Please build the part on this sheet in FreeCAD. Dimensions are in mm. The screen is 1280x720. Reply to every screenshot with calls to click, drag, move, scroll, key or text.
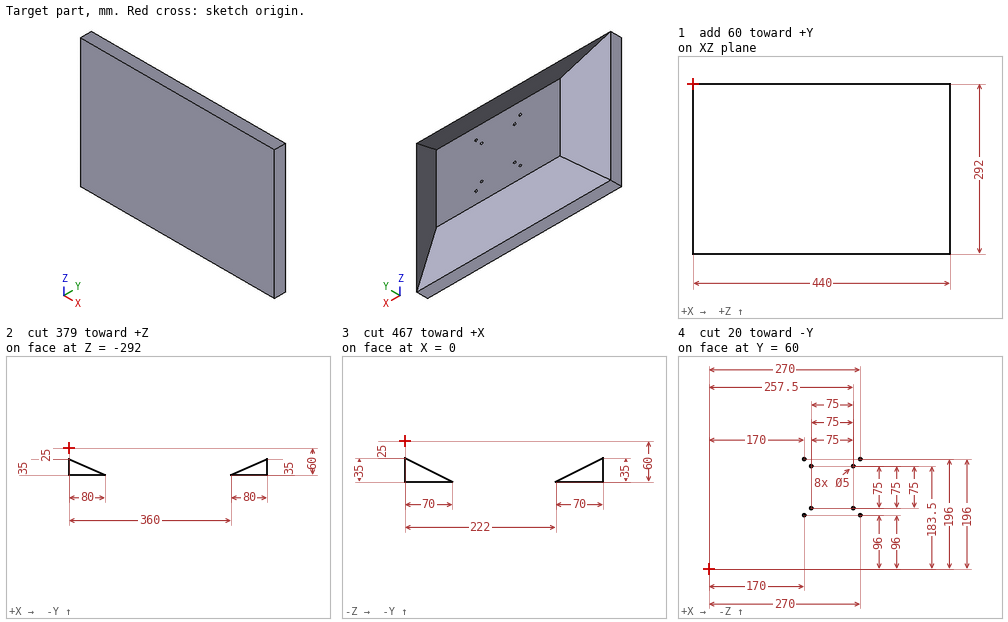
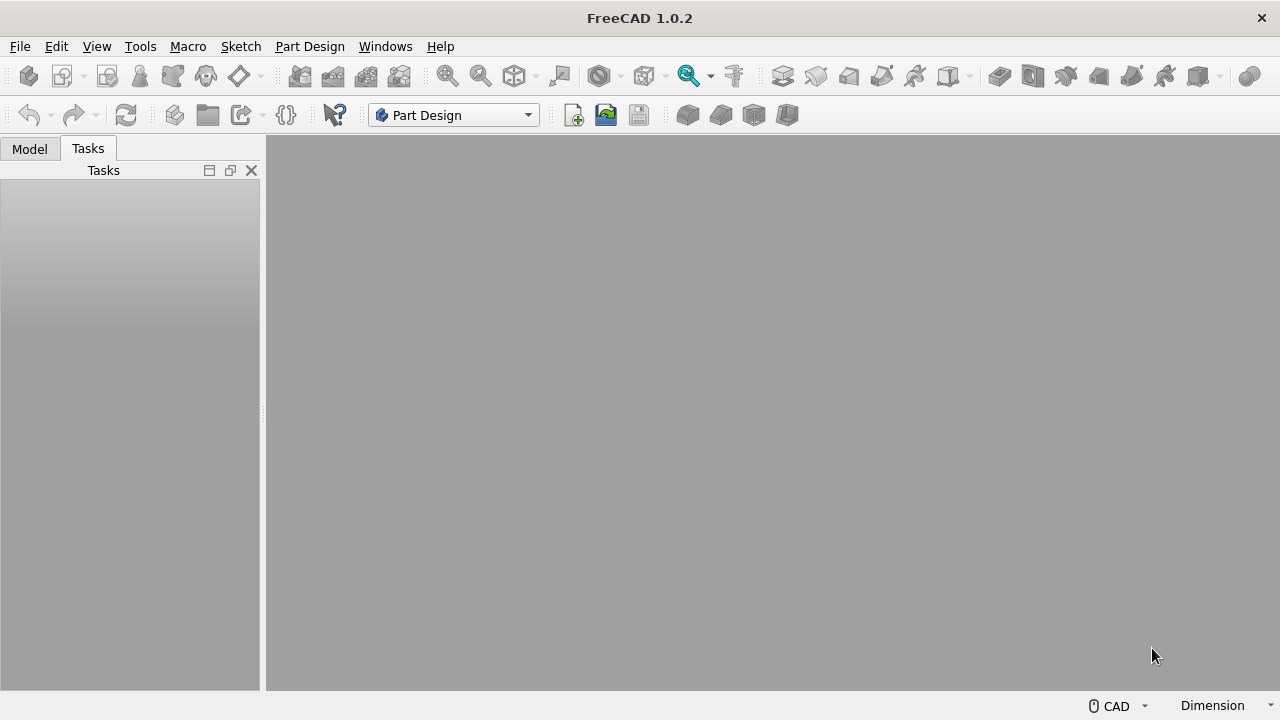
key(ctrl+n)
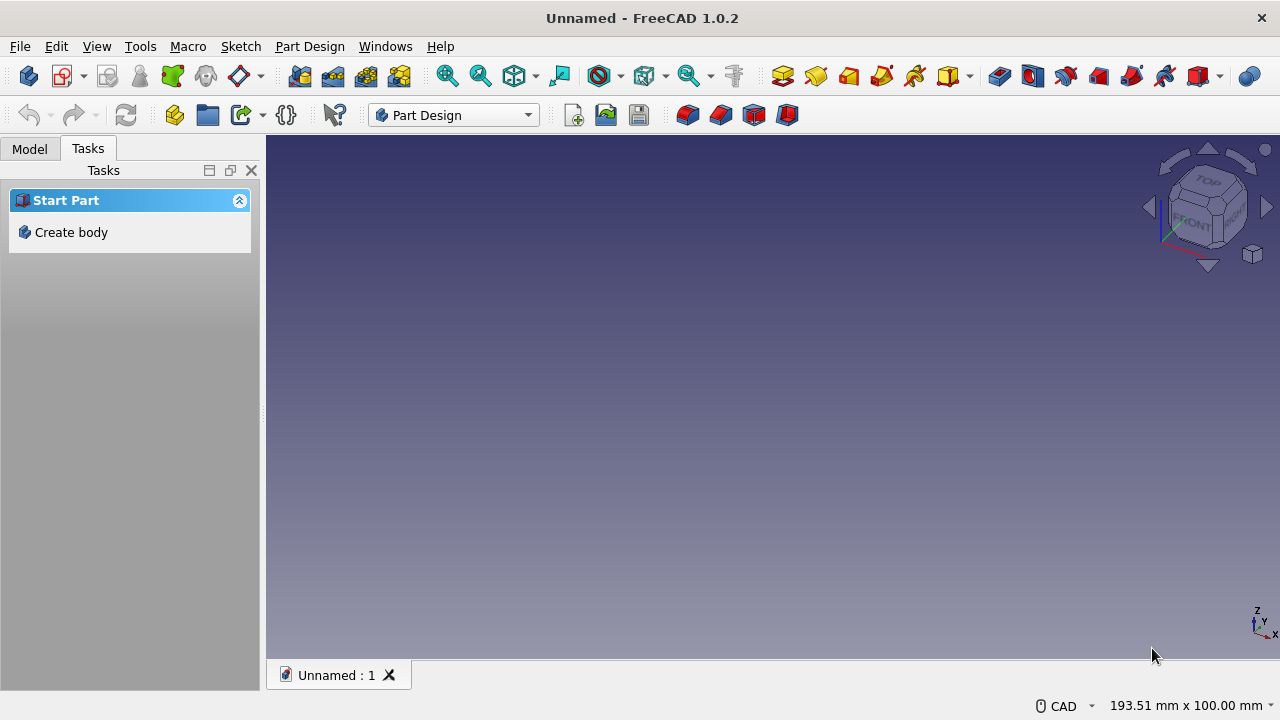
click(62, 76)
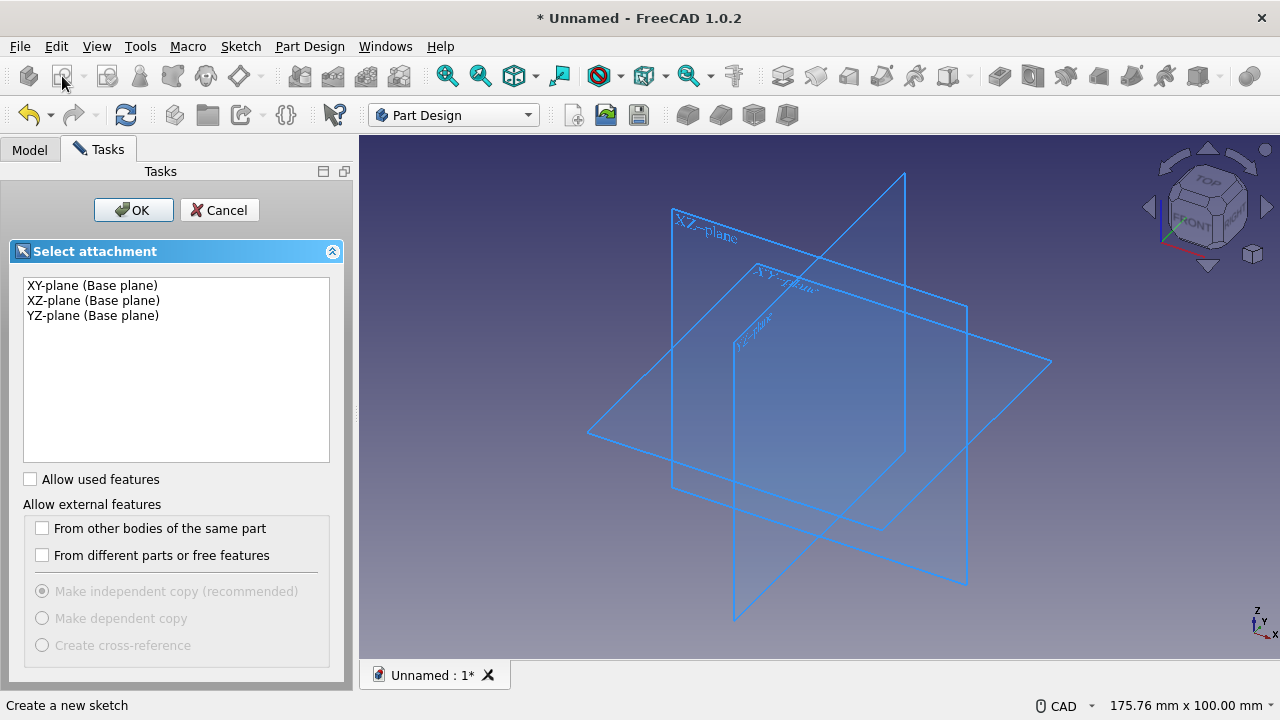
click(84, 300)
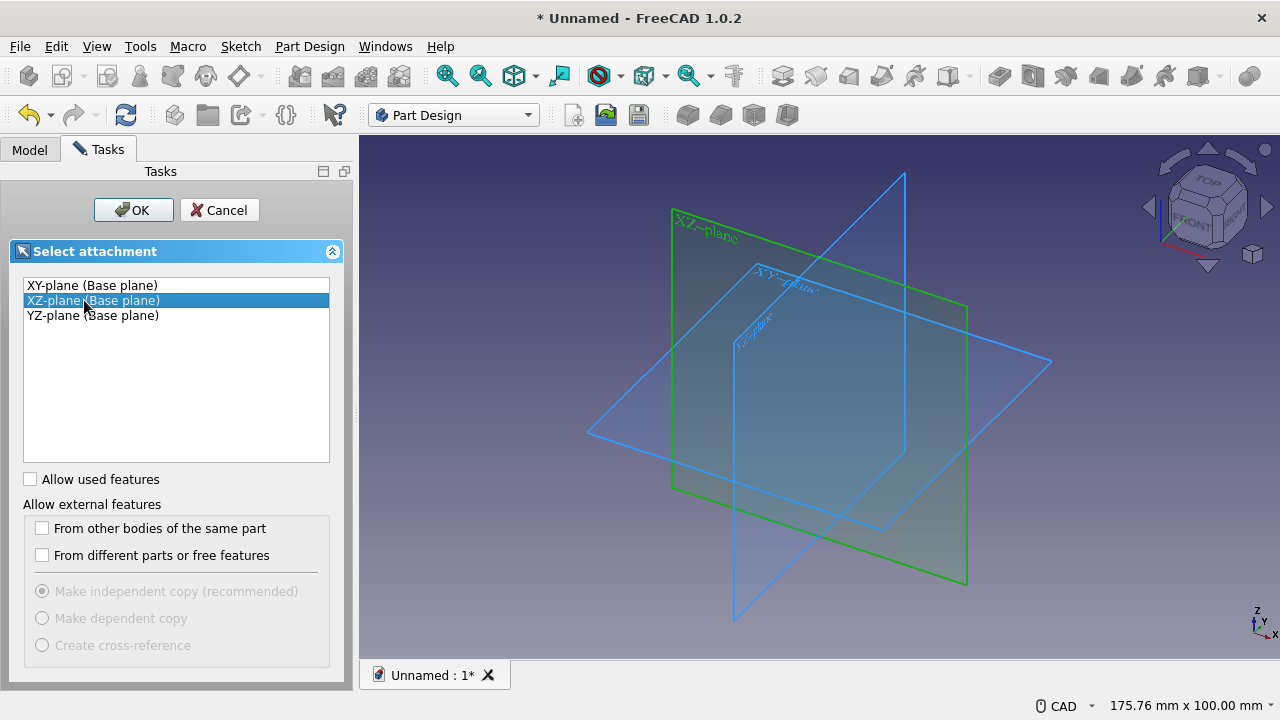
click(134, 210)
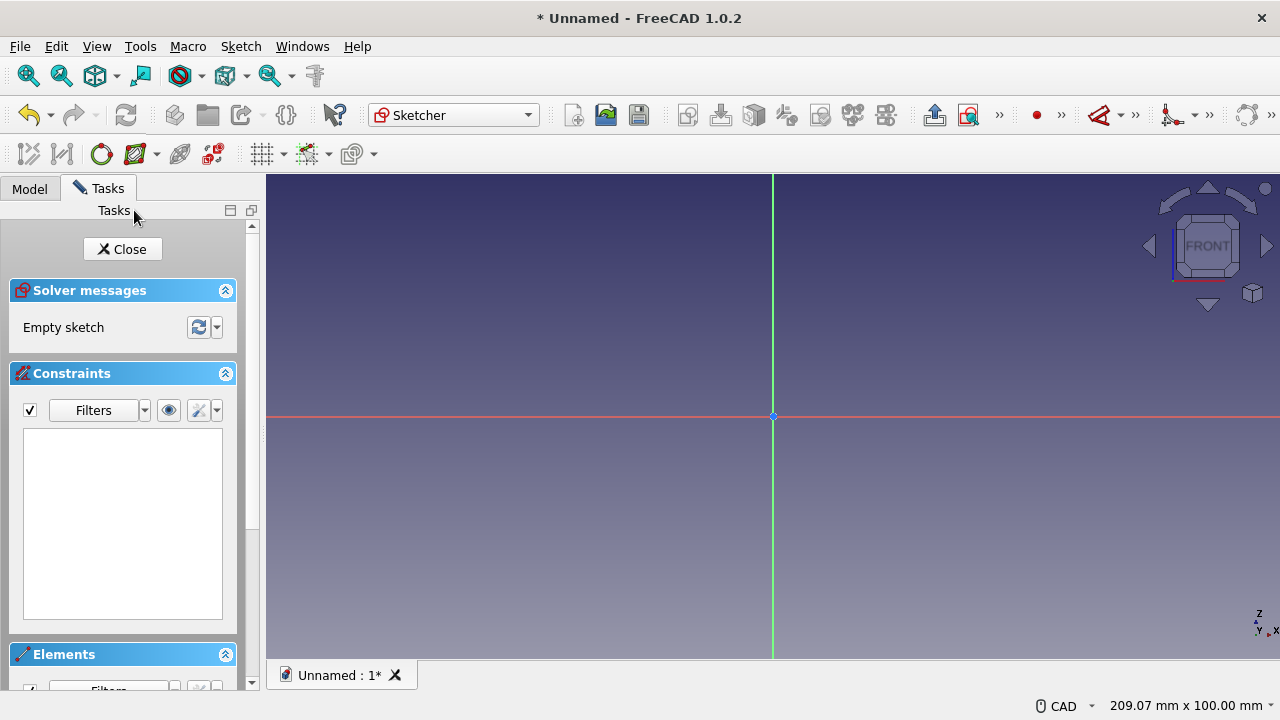
scroll(417, 237, down, 8)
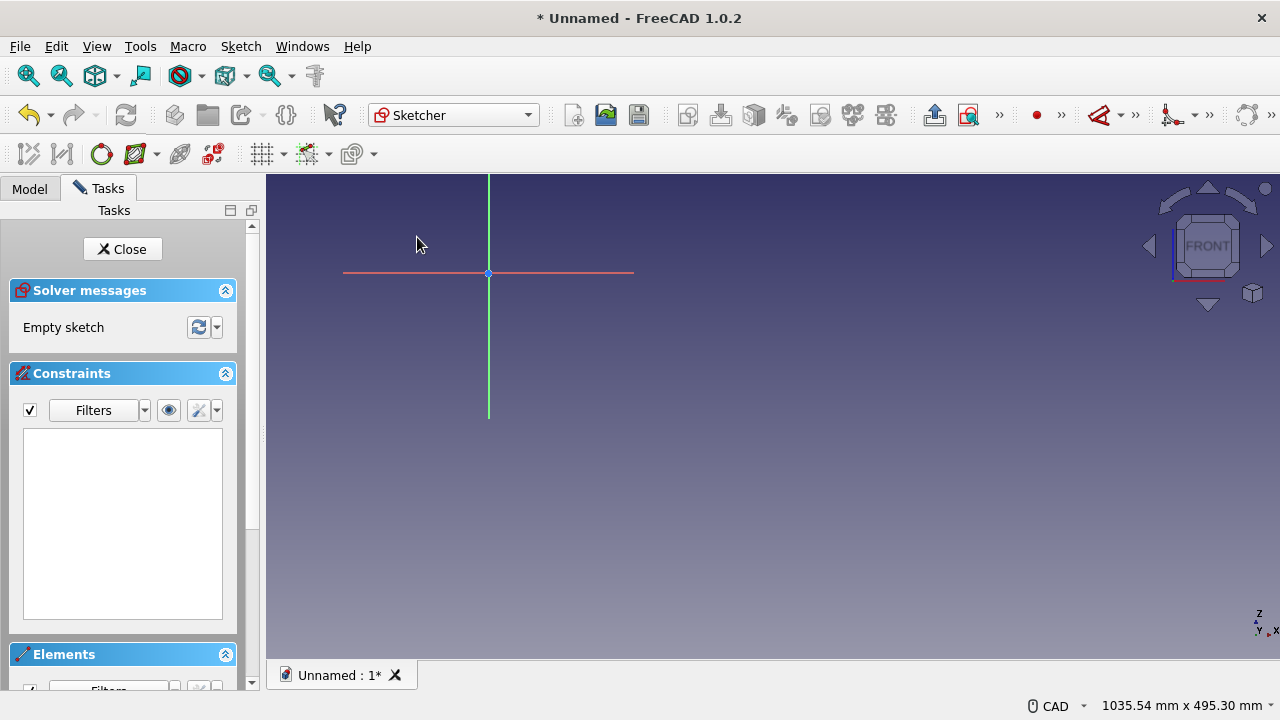
key(g)
key(r)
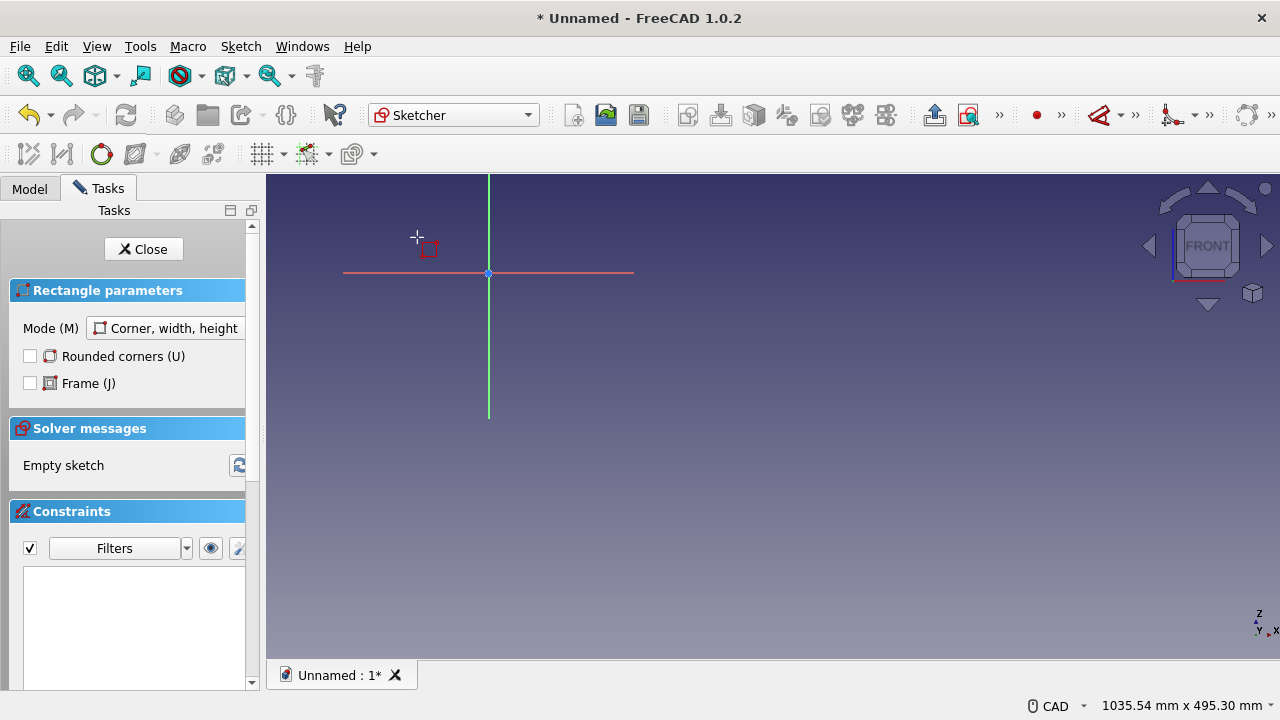
click(489, 273)
move(920, 559)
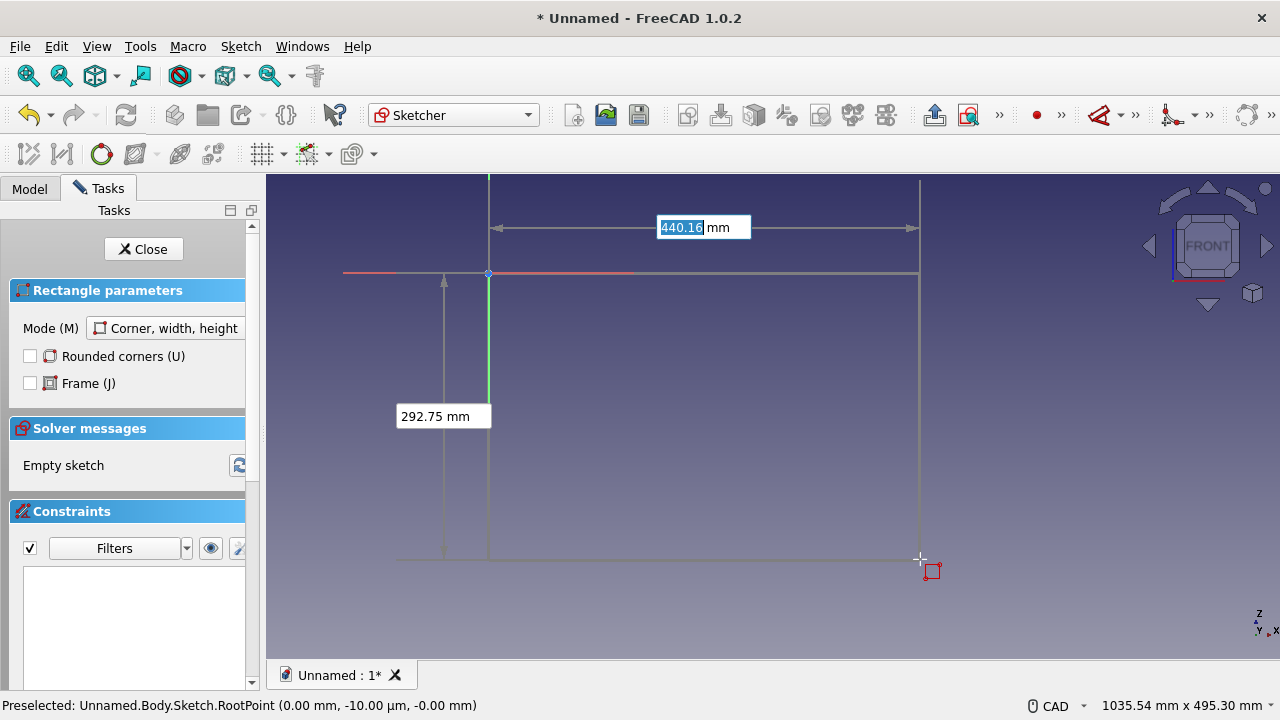
text(440)
key(Tab)
text(292)
key(Return)
key(Escape)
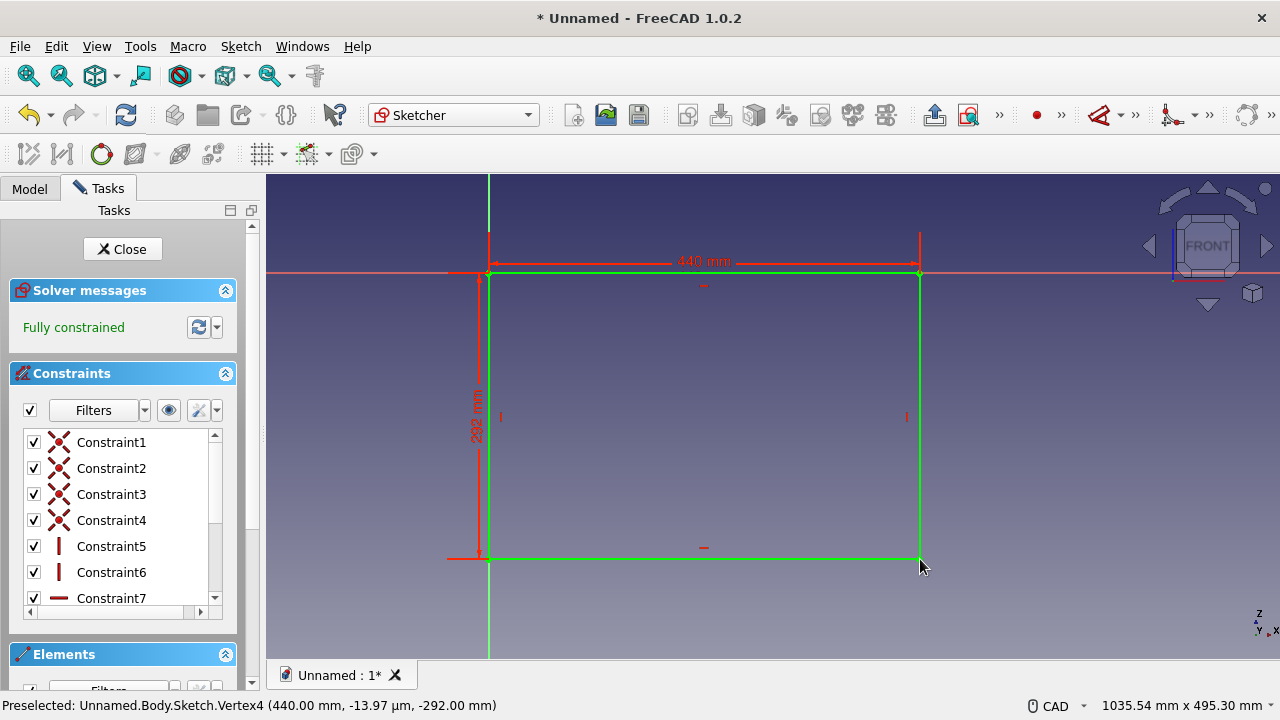
click(123, 249)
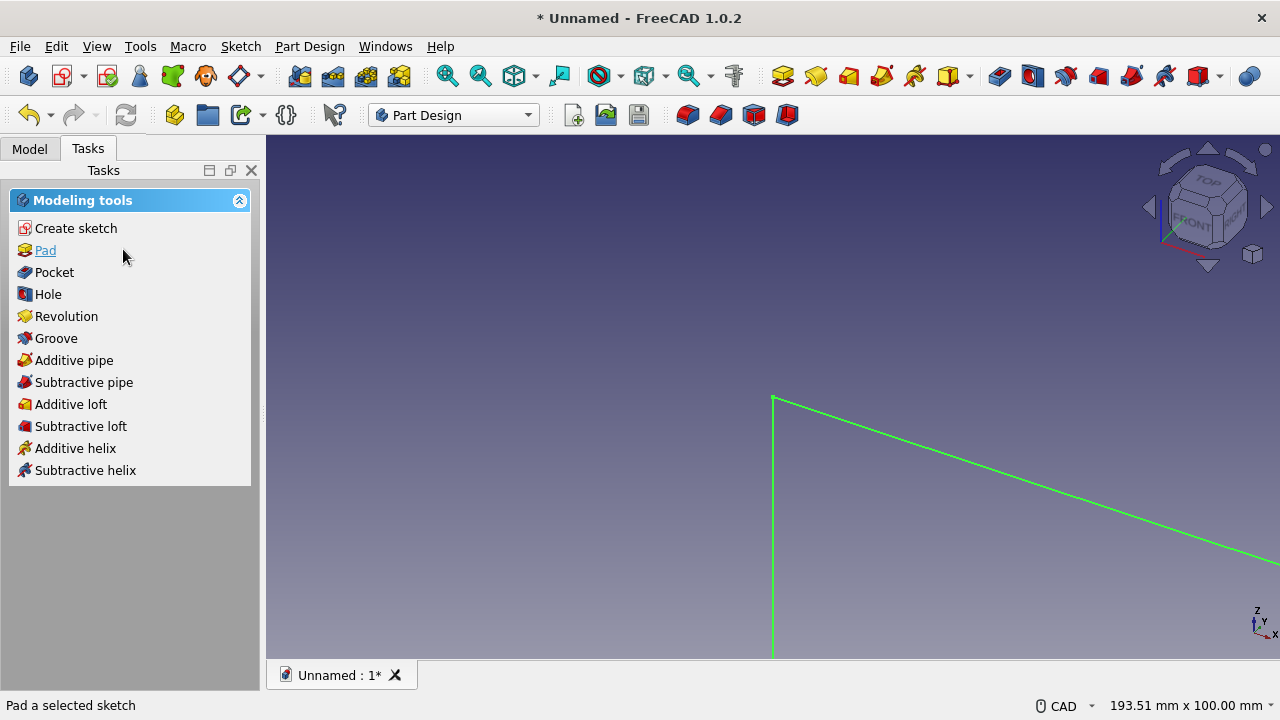
click(783, 76)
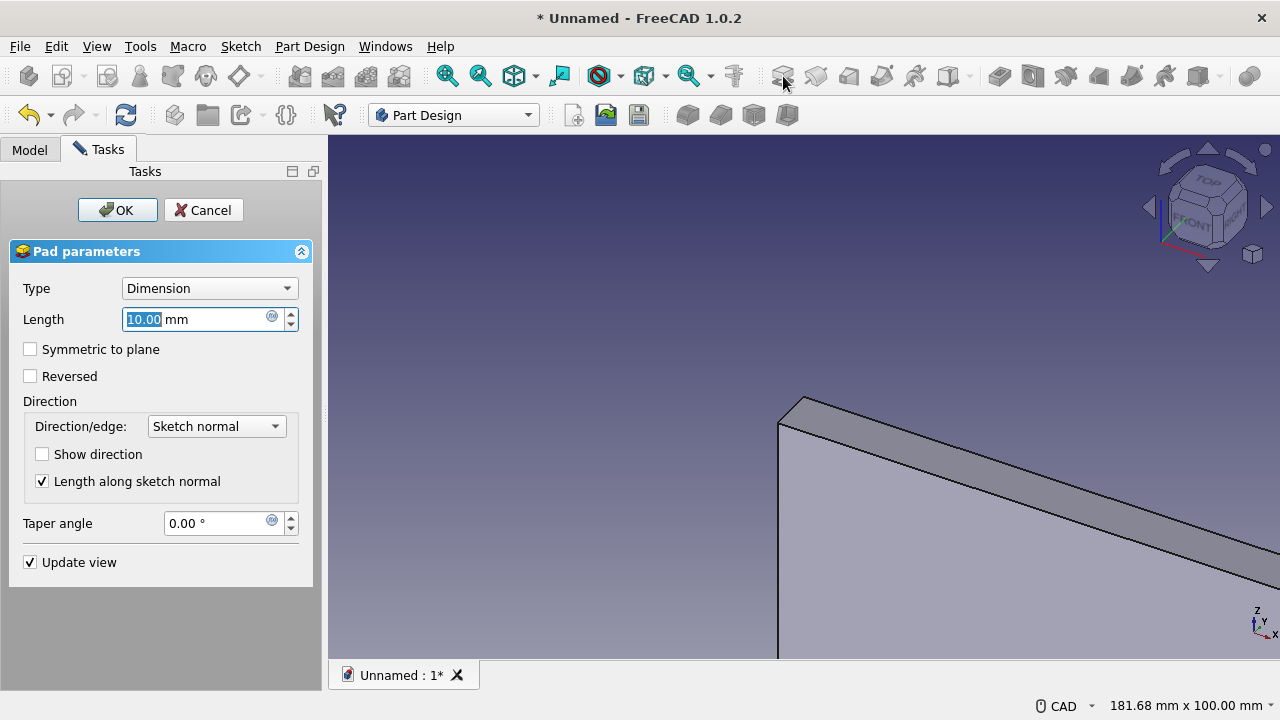
text(60)
key(Tab)